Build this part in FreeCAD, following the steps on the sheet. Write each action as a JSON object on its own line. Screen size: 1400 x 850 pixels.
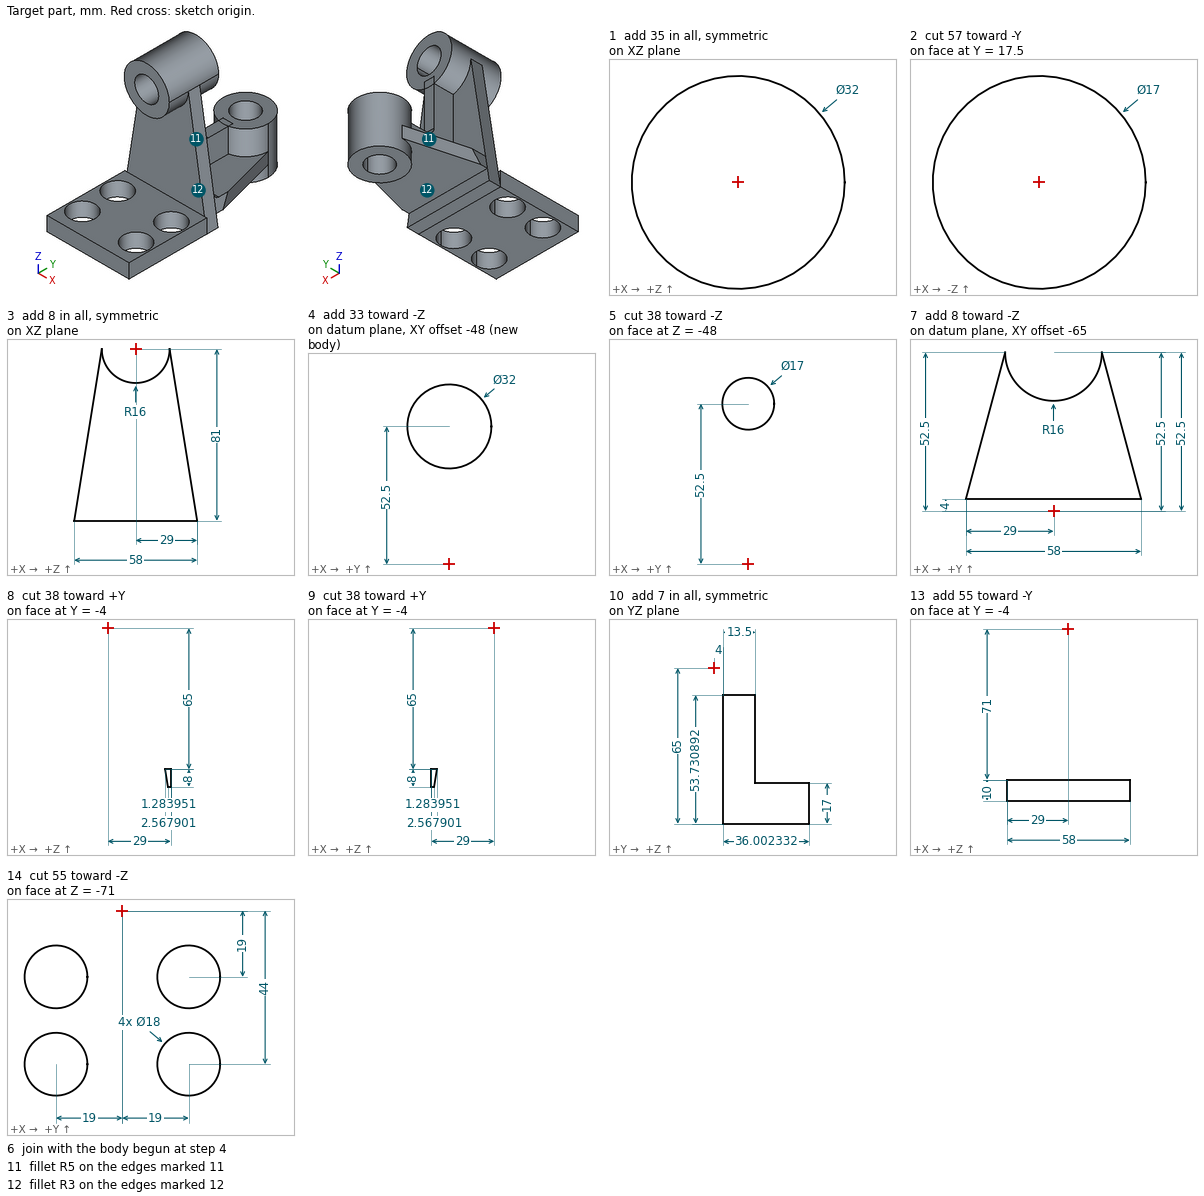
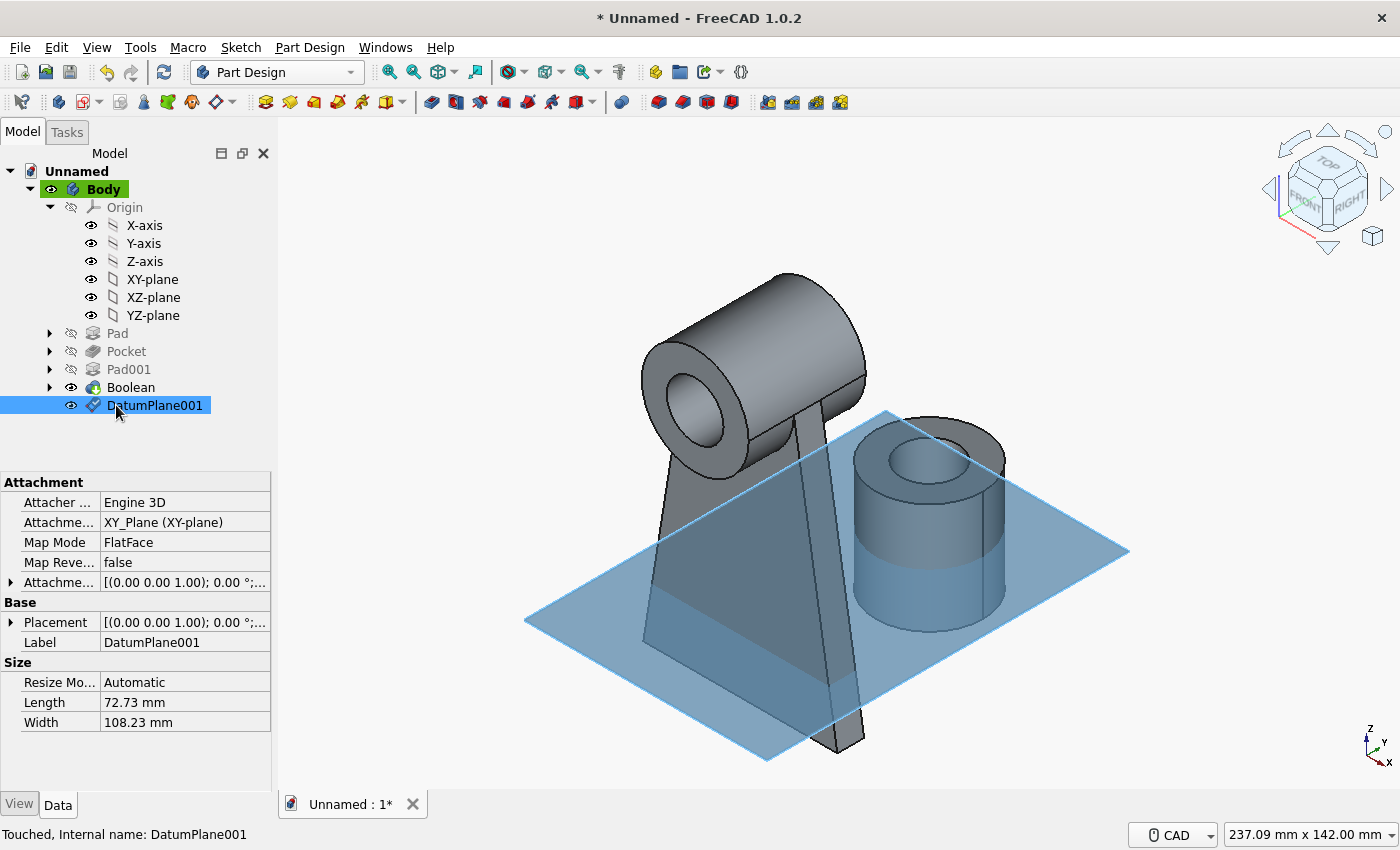
{"action": "left_click", "coordinate": [84, 102]}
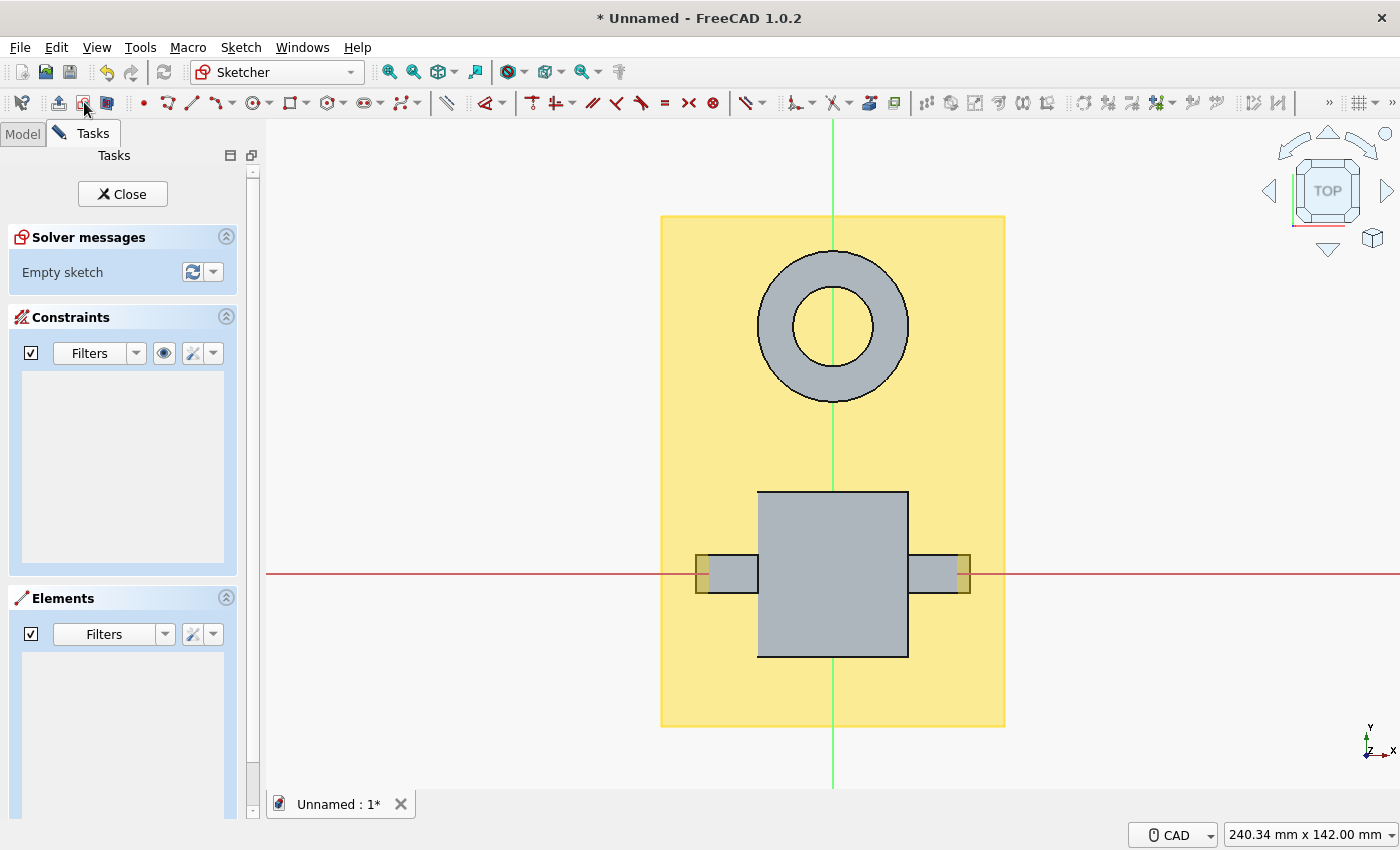
{"action": "key", "text": "q s"}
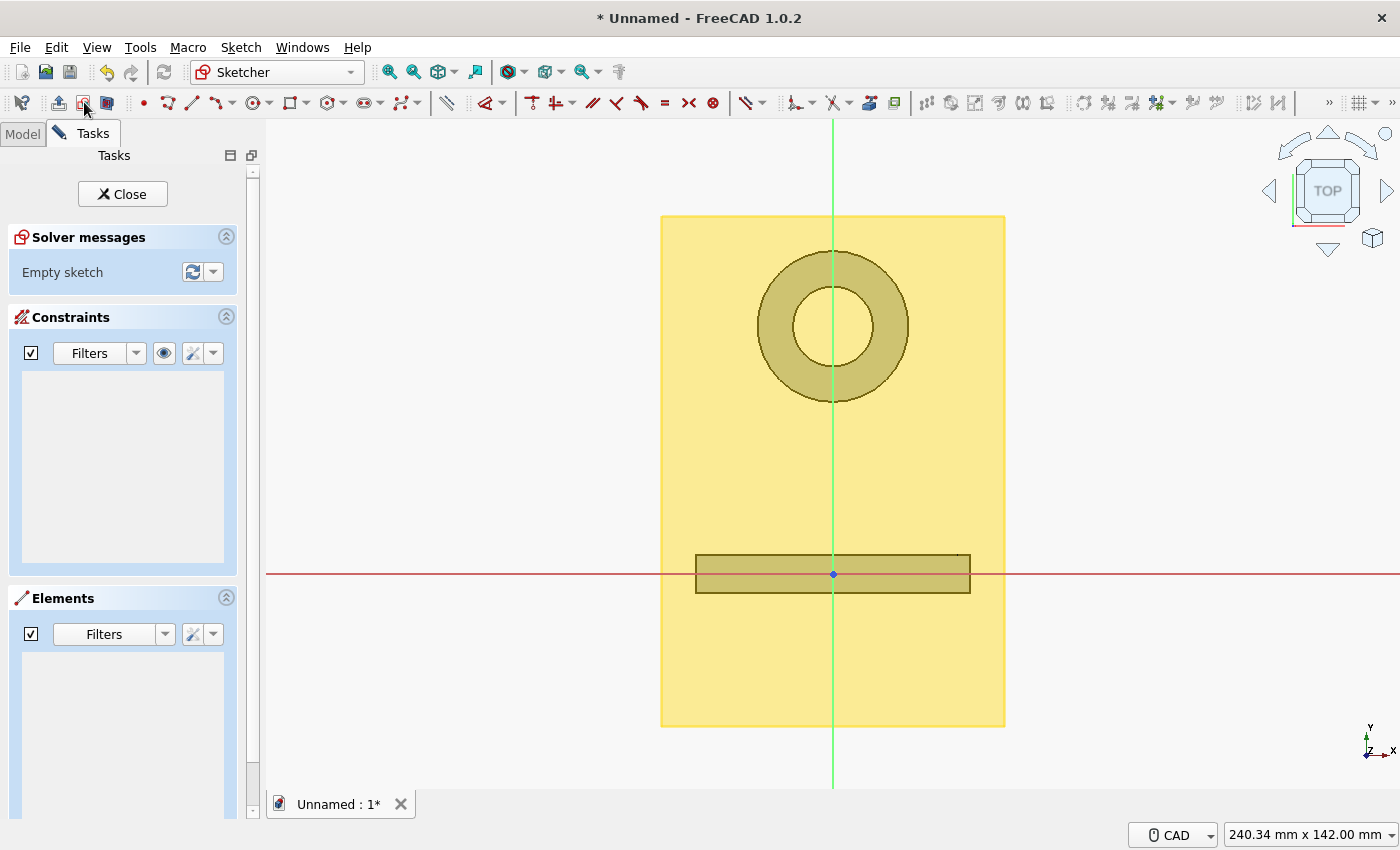
{"action": "scroll", "coordinate": [916, 446], "scroll_direction": "up", "scroll_amount": 3}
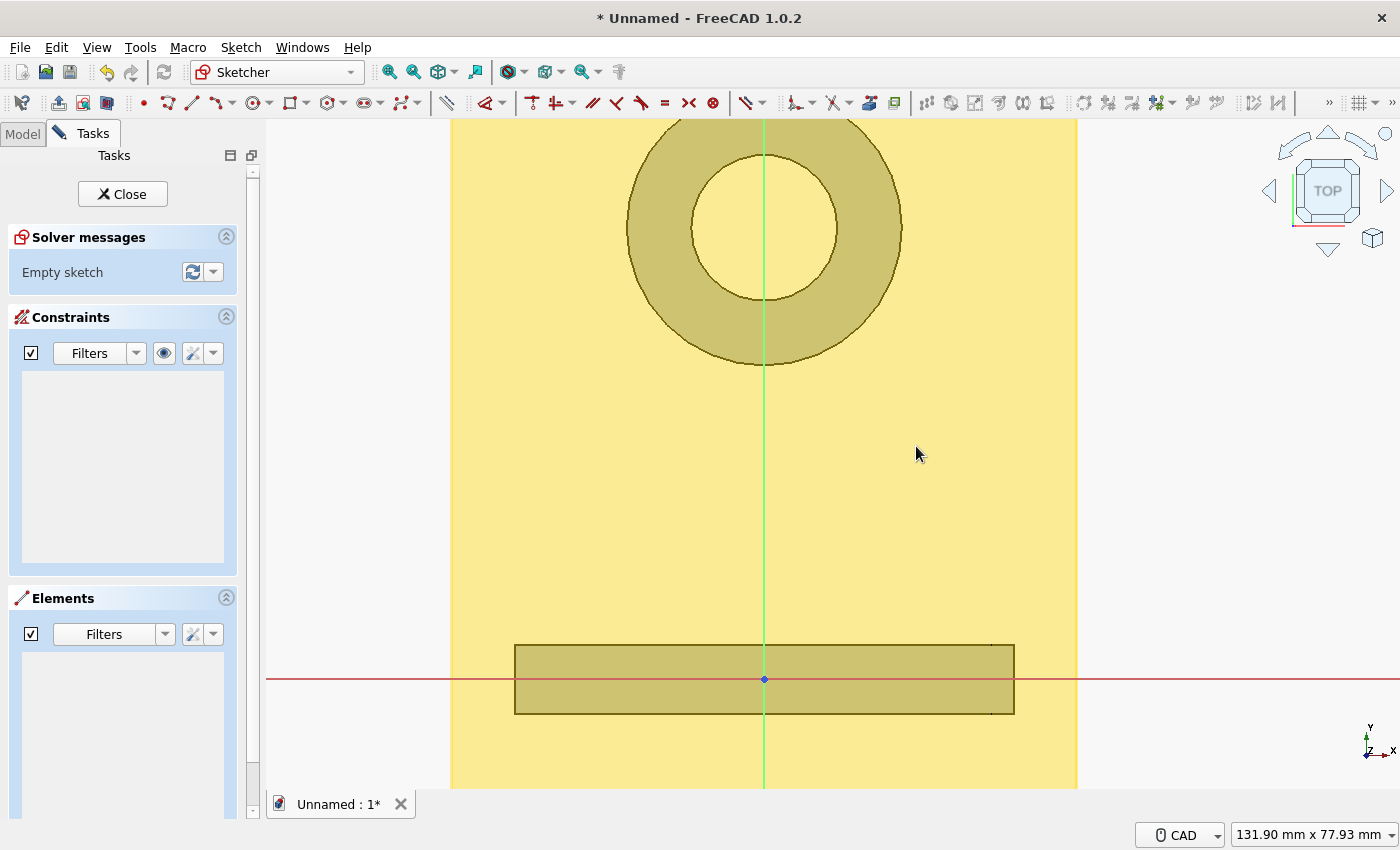
{"action": "left_click", "coordinate": [168, 104]}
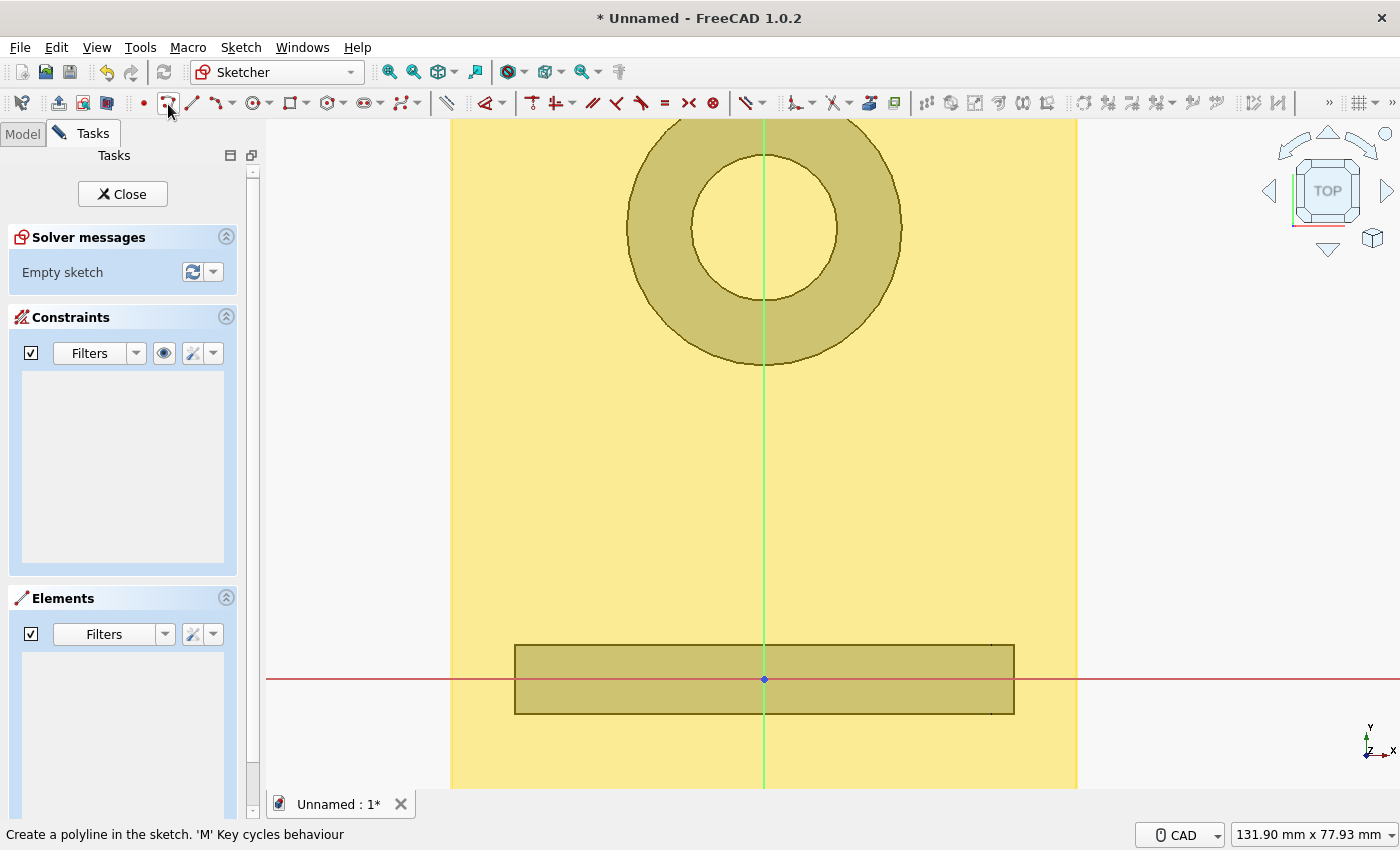
{"action": "left_click", "coordinate": [627, 228]}
{"action": "left_click", "coordinate": [515, 645]}
{"action": "left_click", "coordinate": [1014, 645]}
{"action": "left_click", "coordinate": [902, 228]}
{"action": "right_click", "coordinate": [902, 228]}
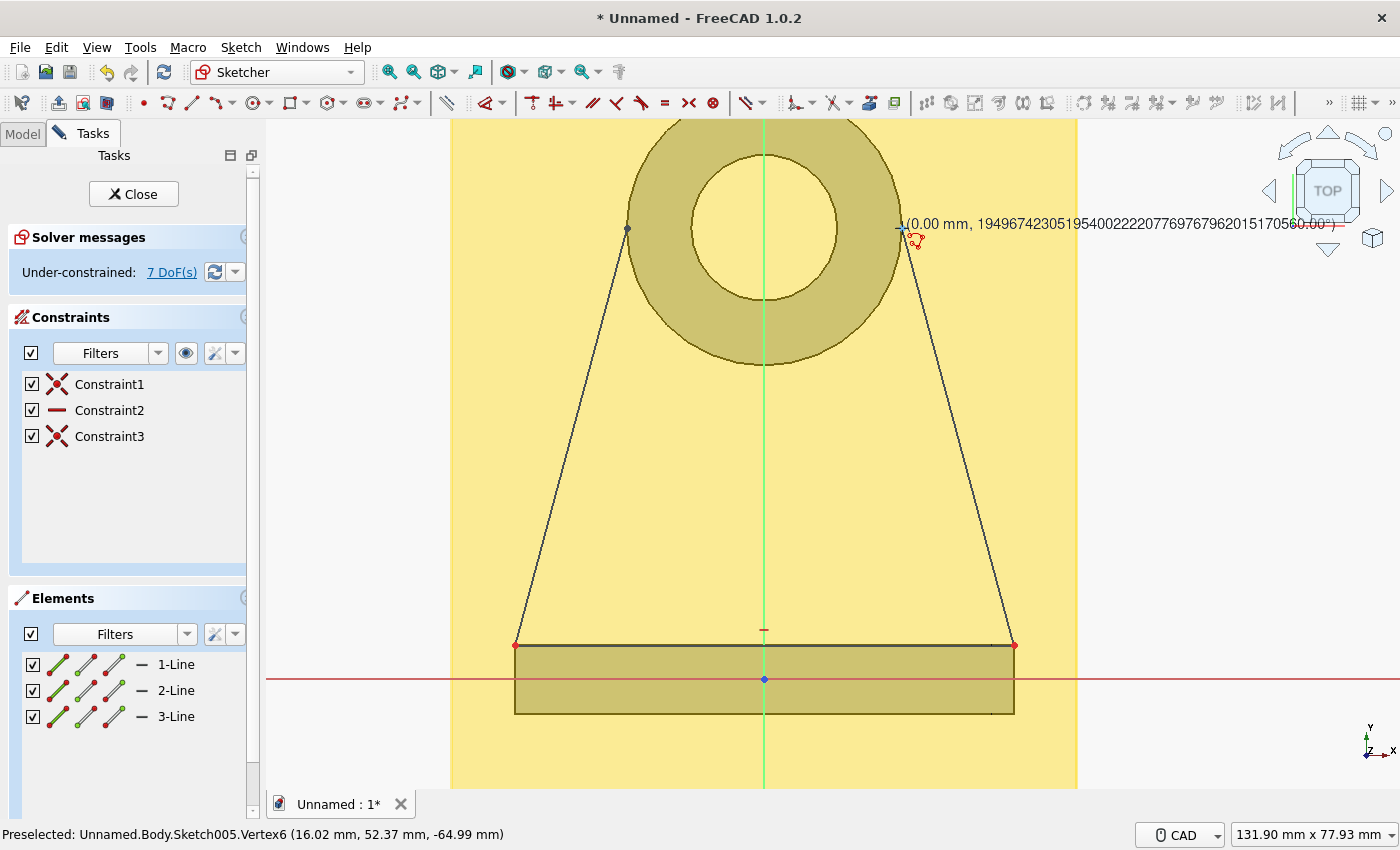
{"action": "key", "text": "g 3 a"}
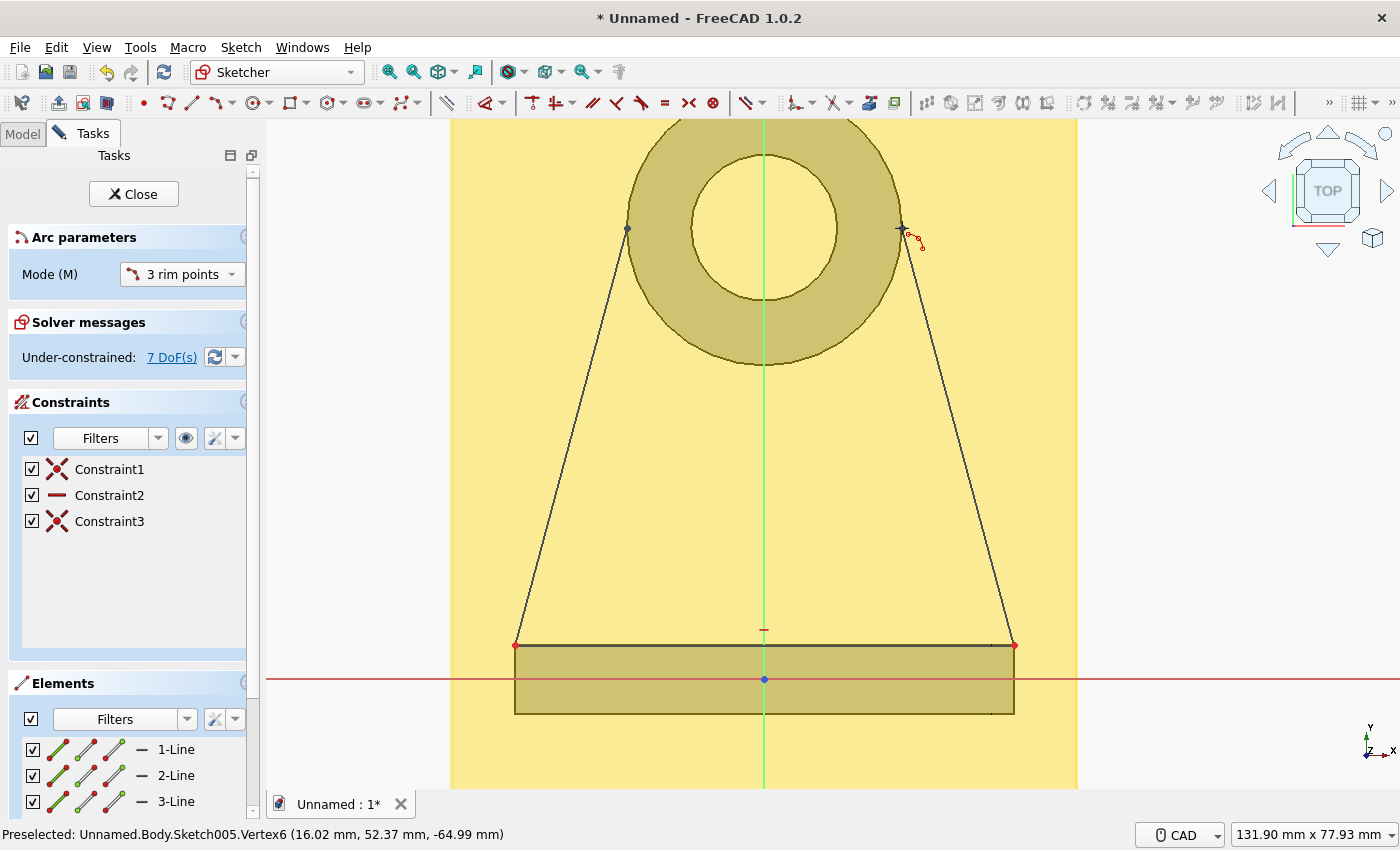
{"action": "left_click", "coordinate": [902, 229]}
{"action": "left_click", "coordinate": [627, 229]}
{"action": "left_click", "coordinate": [722, 359]}
{"action": "key", "text": "Escape"}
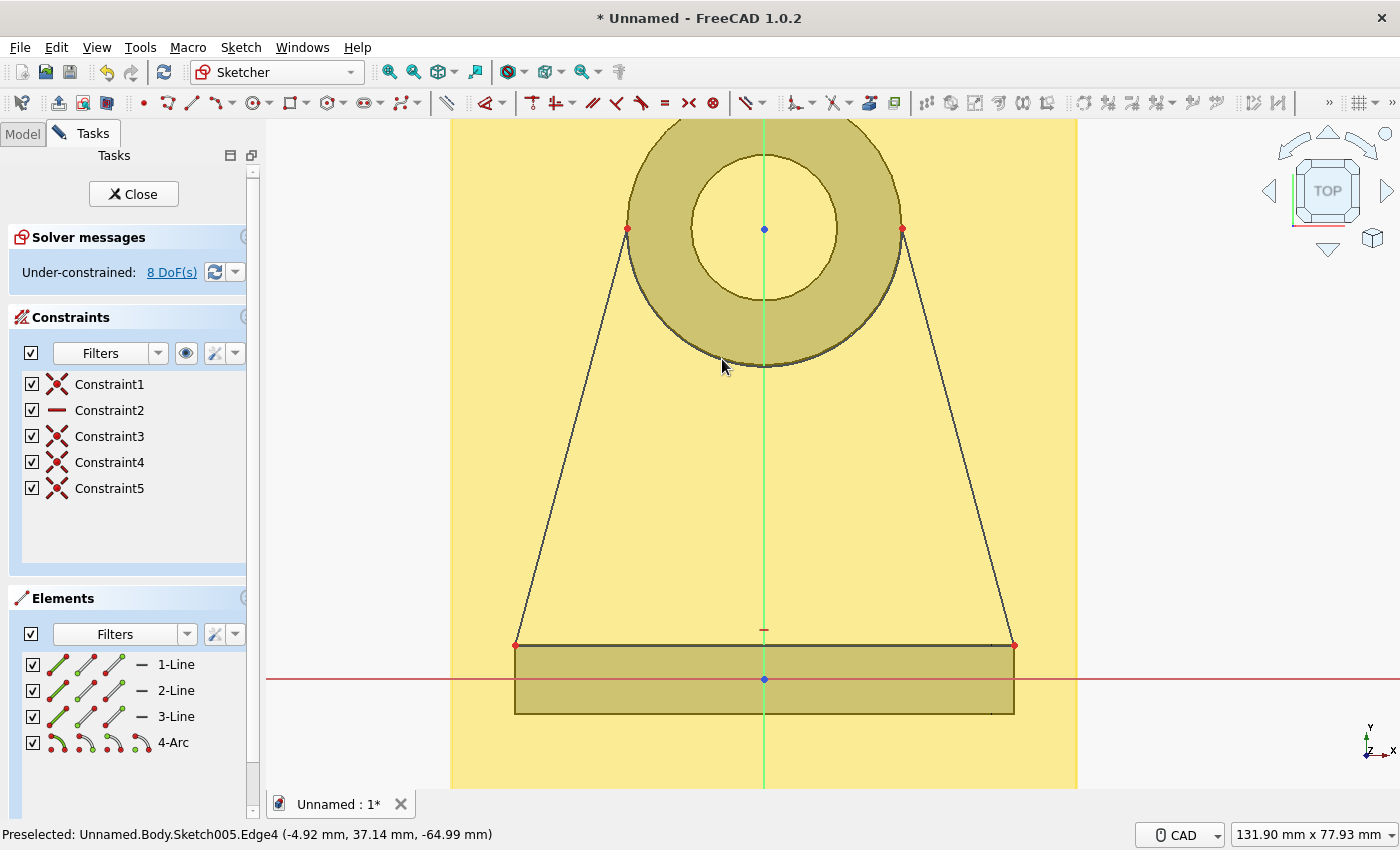
{"action": "left_click", "coordinate": [765, 229]}